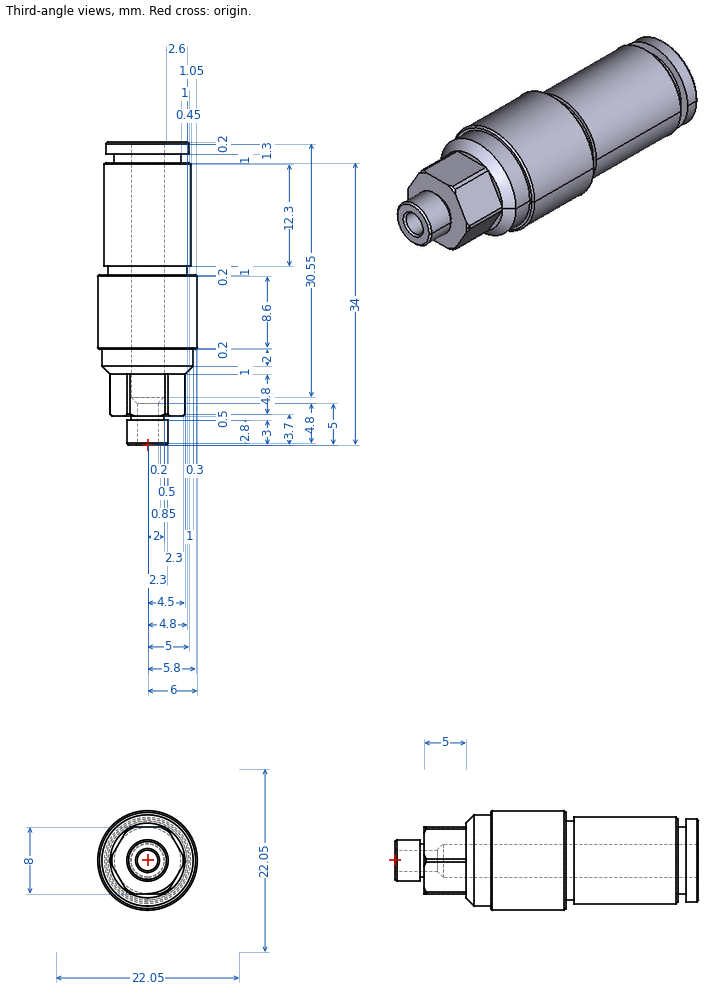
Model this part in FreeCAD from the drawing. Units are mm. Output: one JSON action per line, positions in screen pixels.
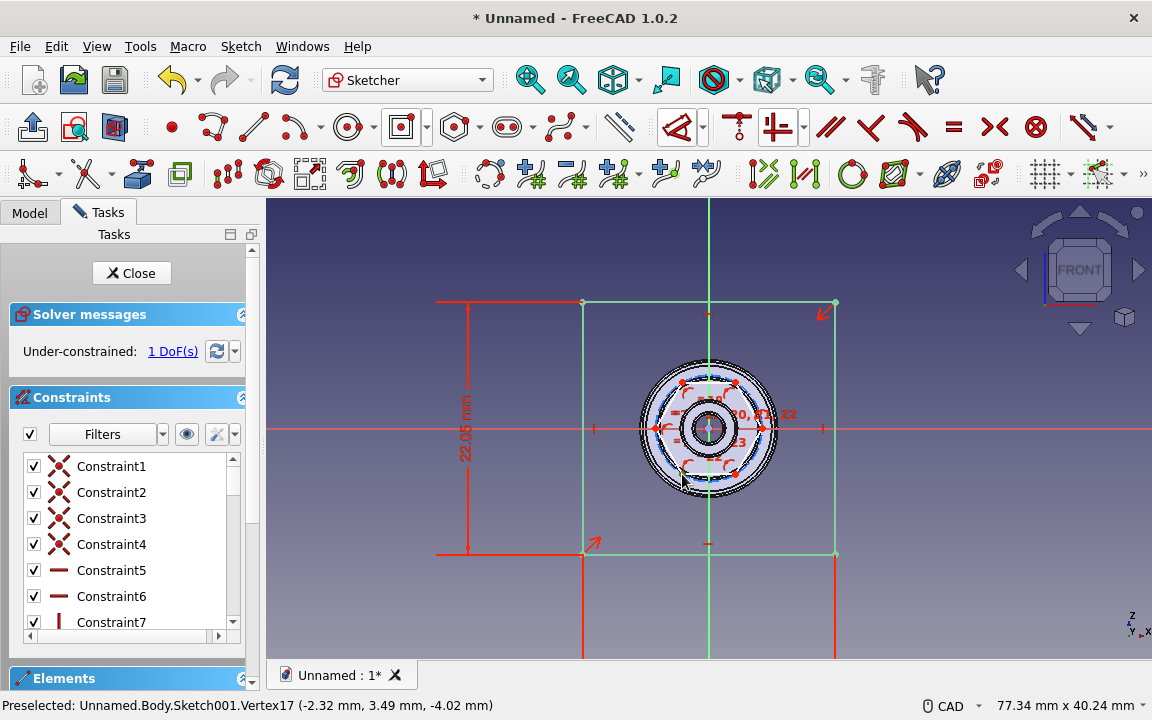
{"action": "left_click", "coordinate": [735, 383]}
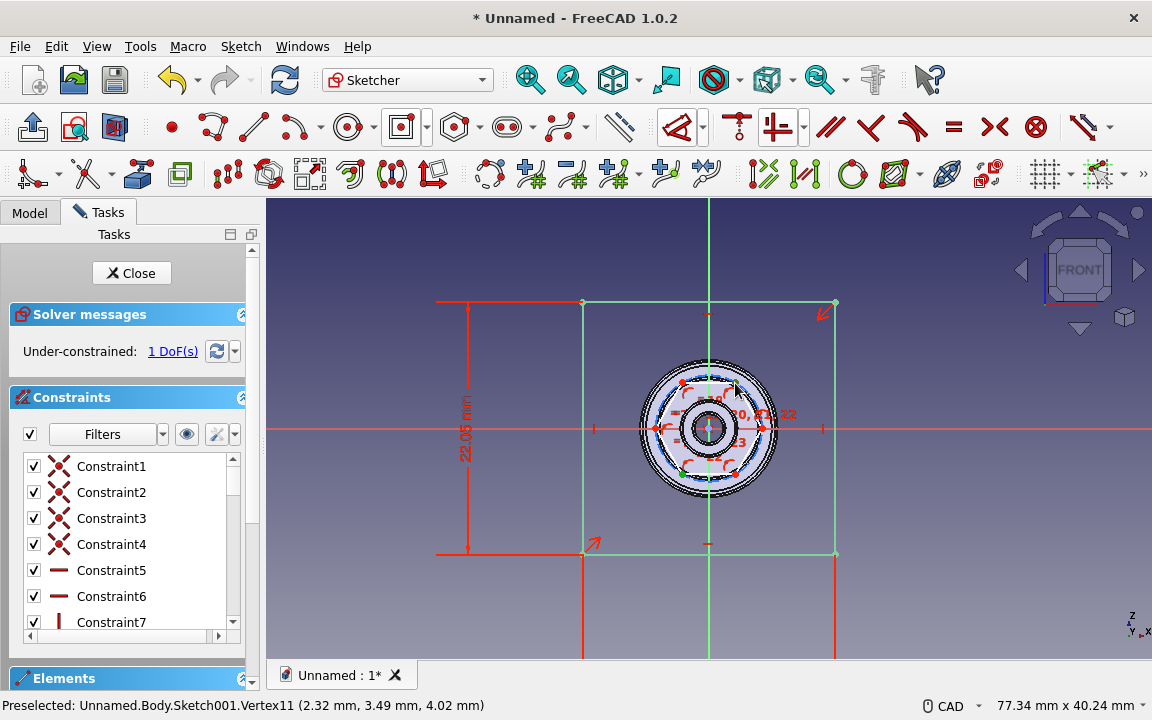
{"action": "key", "text": "i"}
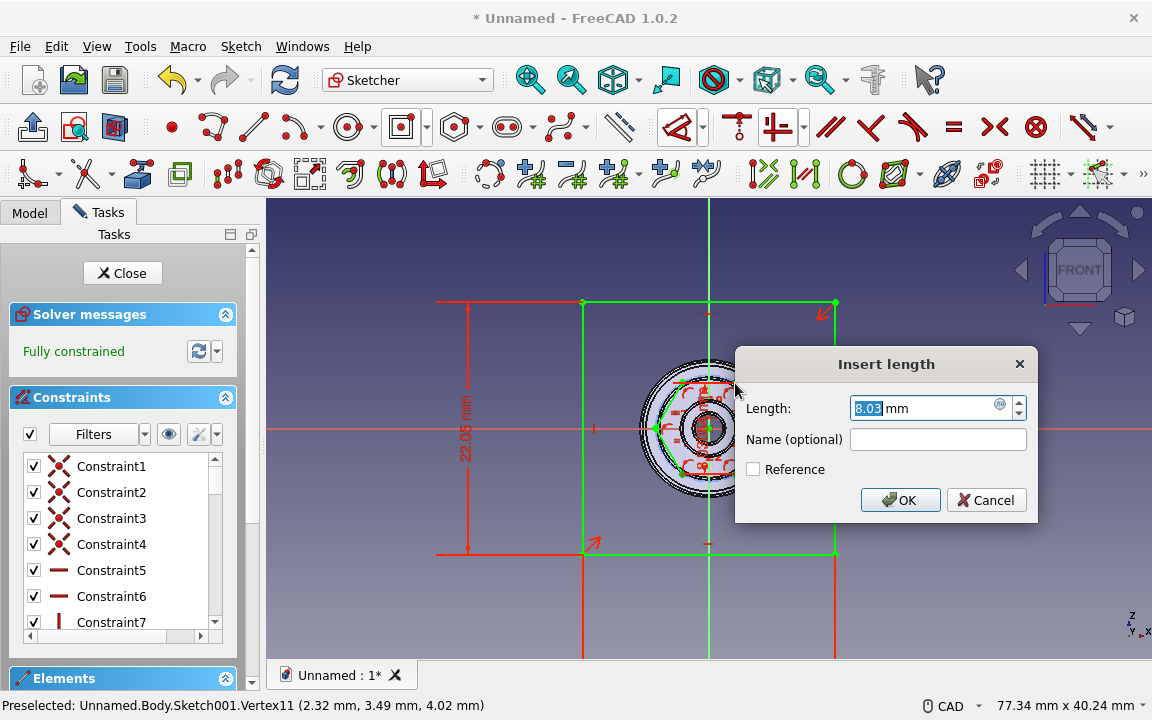
{"action": "type", "text": "8"}
{"action": "key", "text": "Return"}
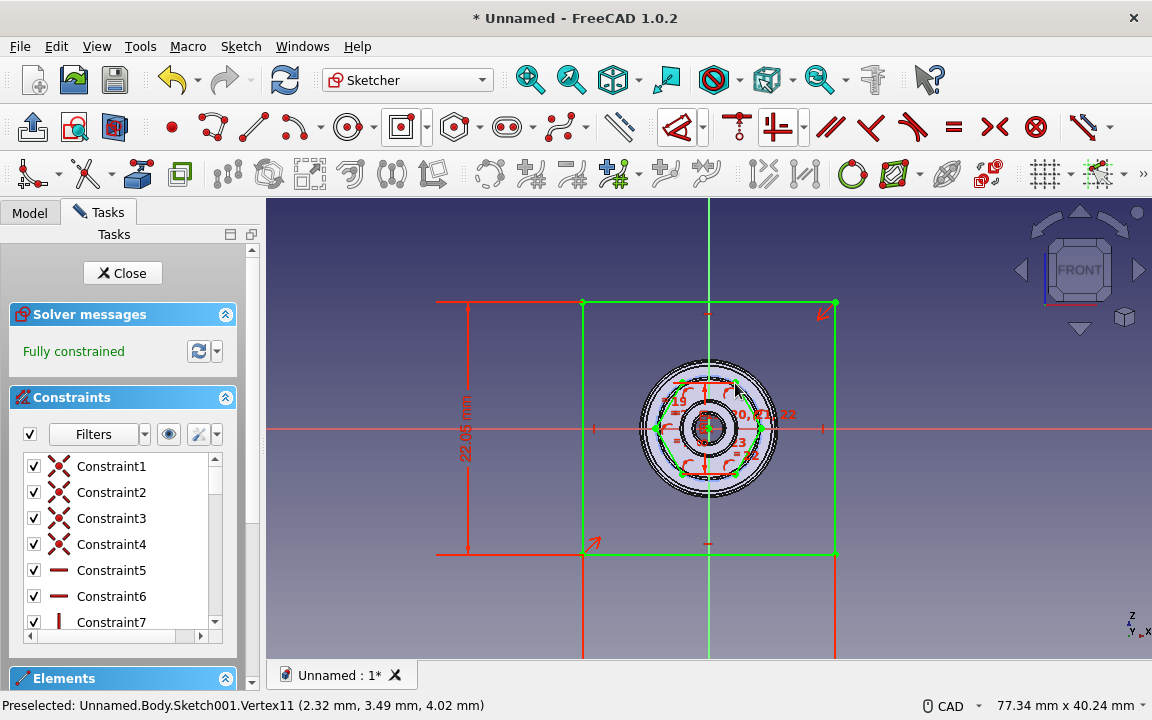
{"action": "left_click", "coordinate": [123, 273]}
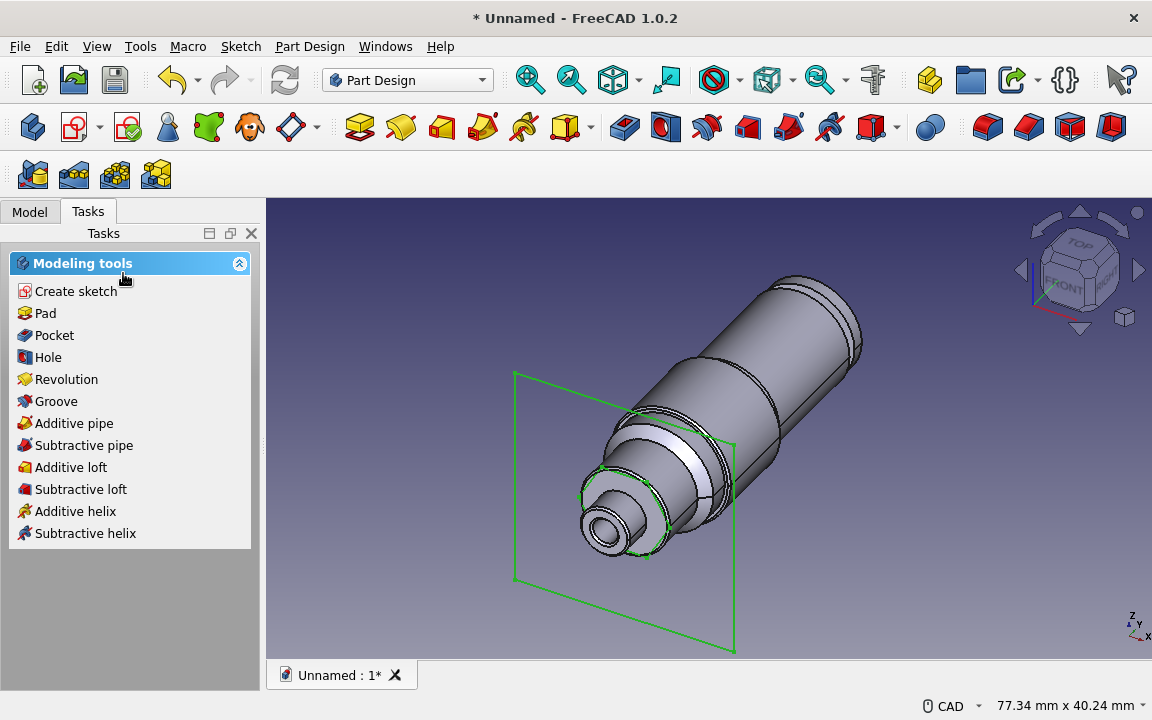
{"action": "left_click", "coordinate": [625, 128]}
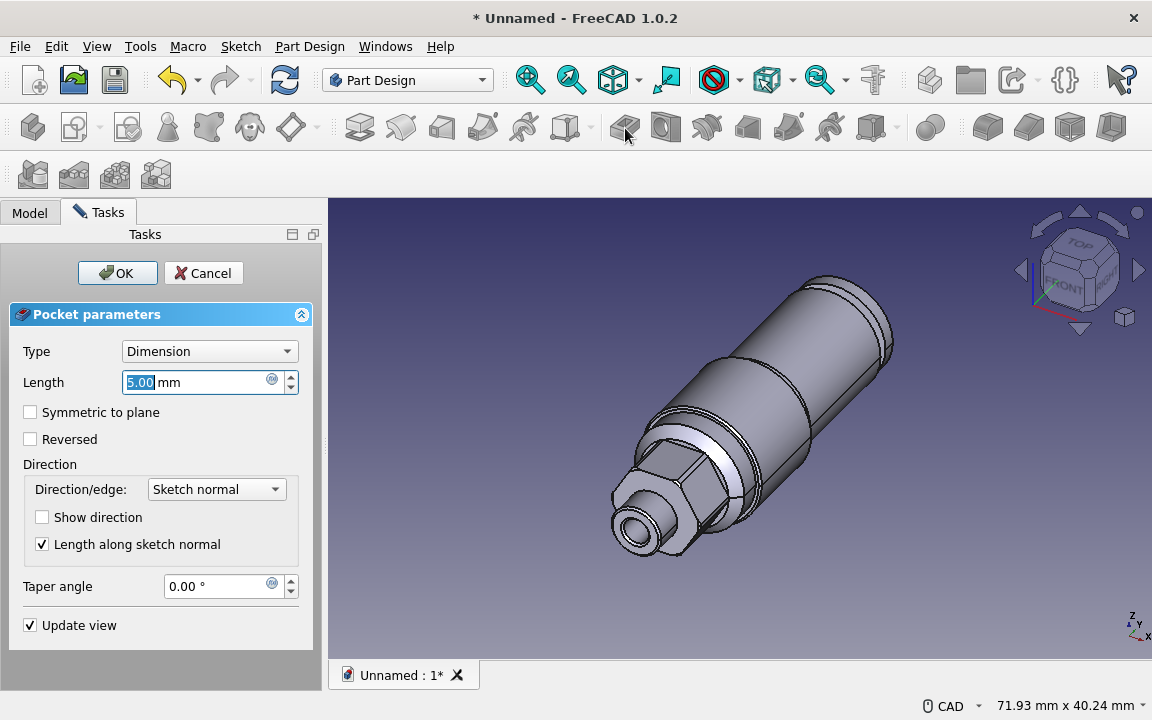
{"action": "type", "text": "5"}
{"action": "key", "text": "Tab"}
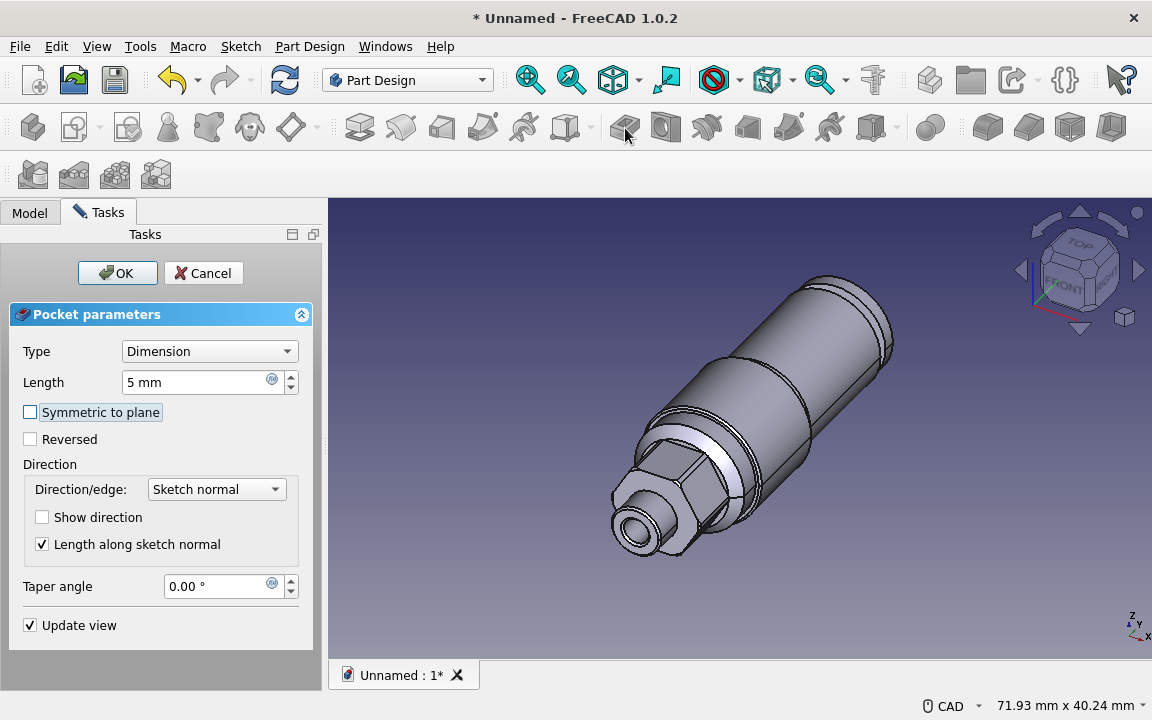
{"action": "left_click", "coordinate": [118, 273]}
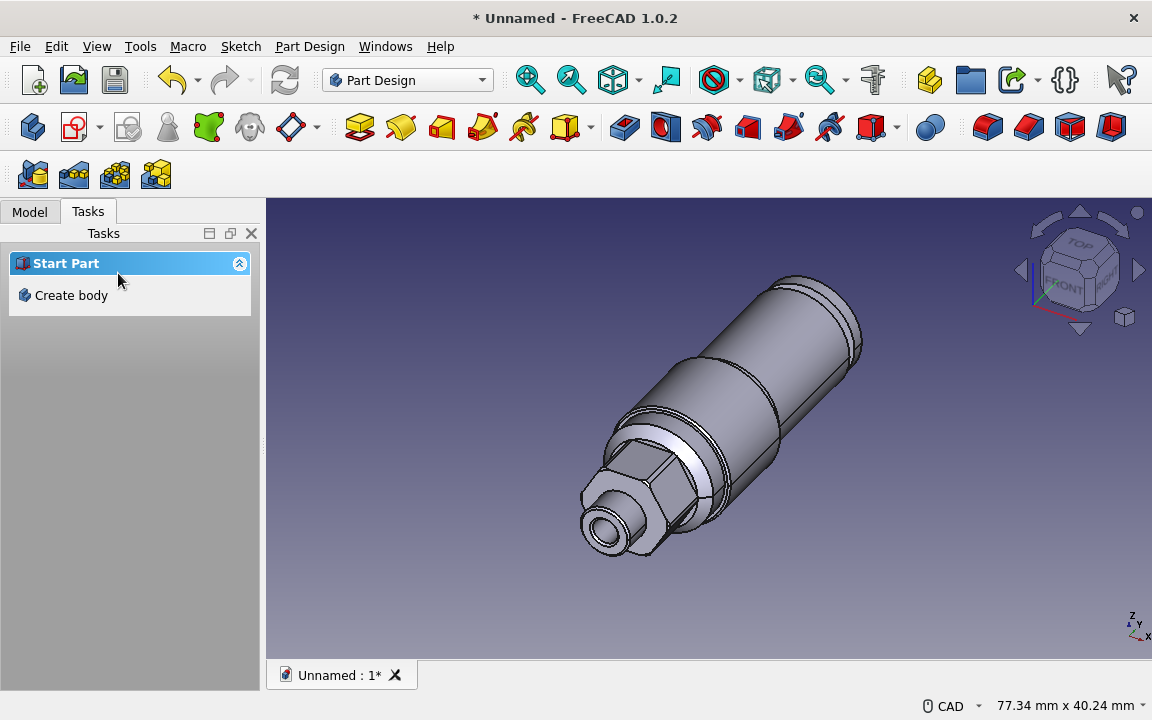
{"action": "key", "text": "0"}